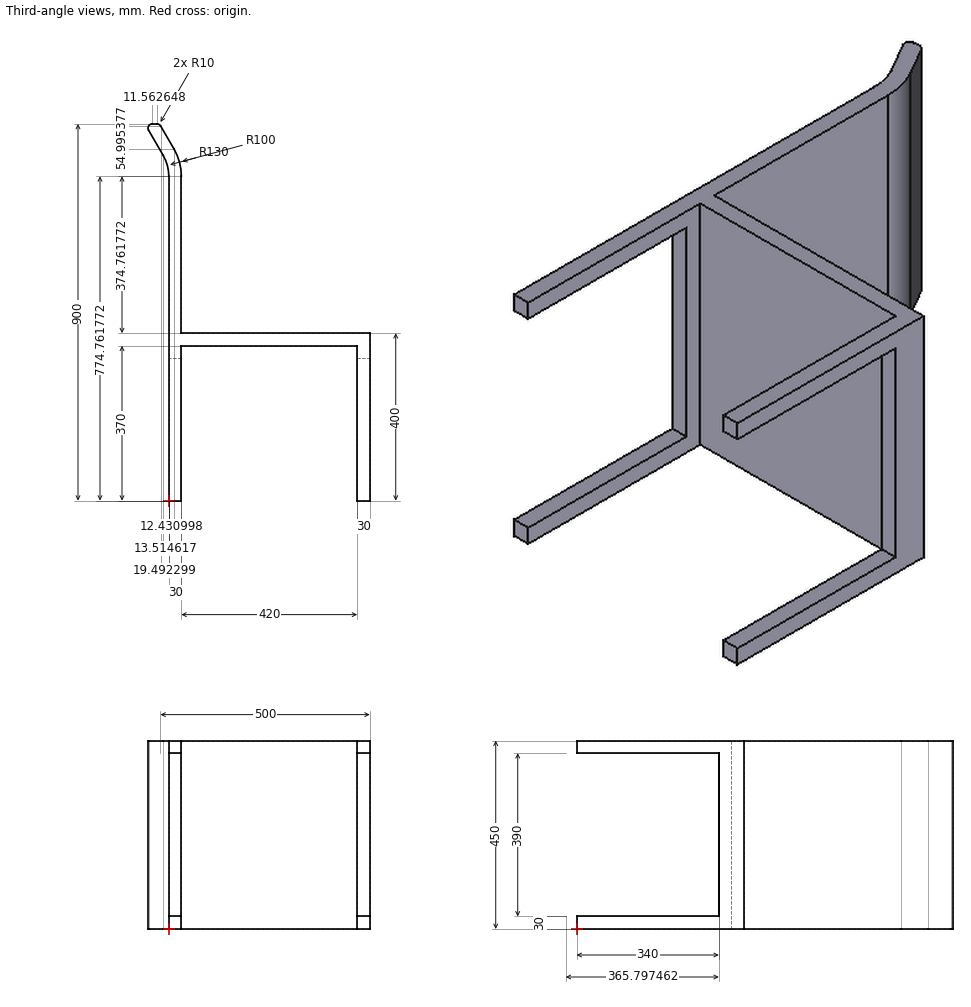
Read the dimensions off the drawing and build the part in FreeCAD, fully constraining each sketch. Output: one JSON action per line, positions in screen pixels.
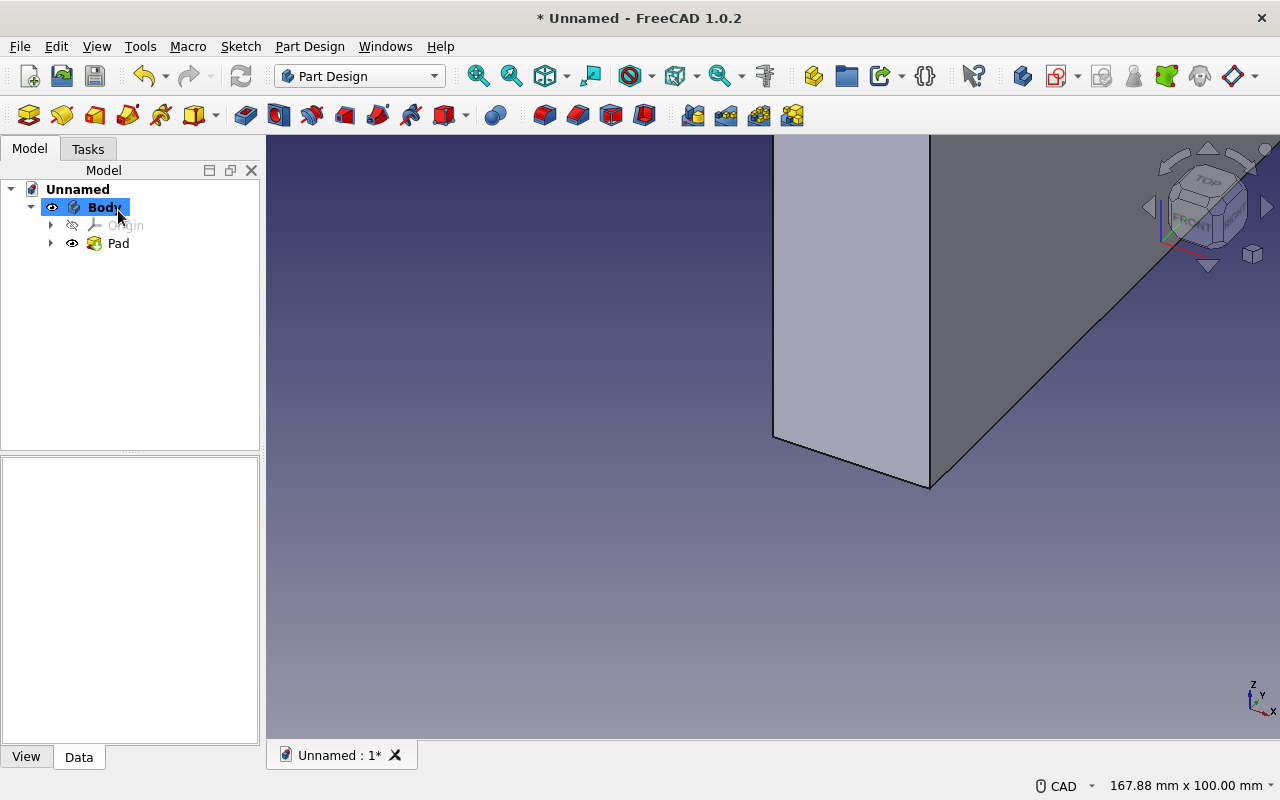
{"action": "key", "text": "v f"}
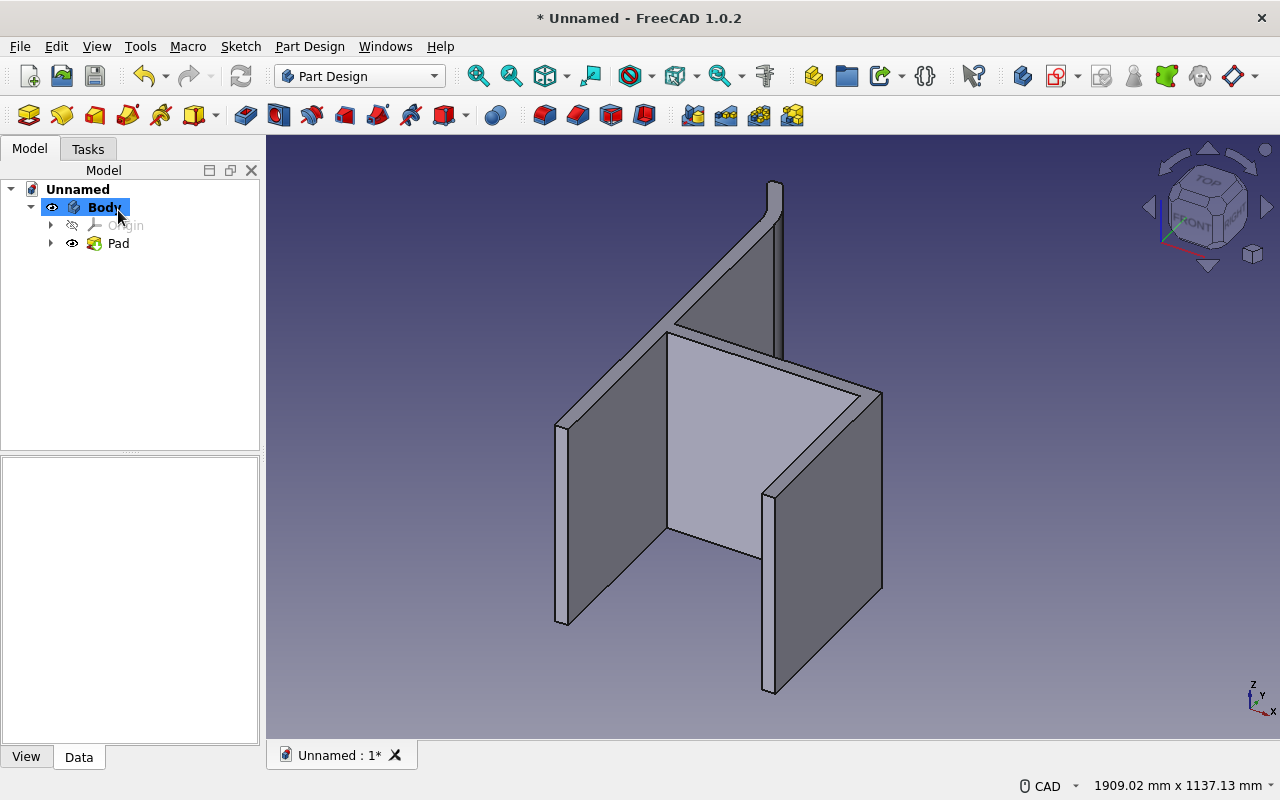
{"action": "left_click", "coordinate": [828, 542]}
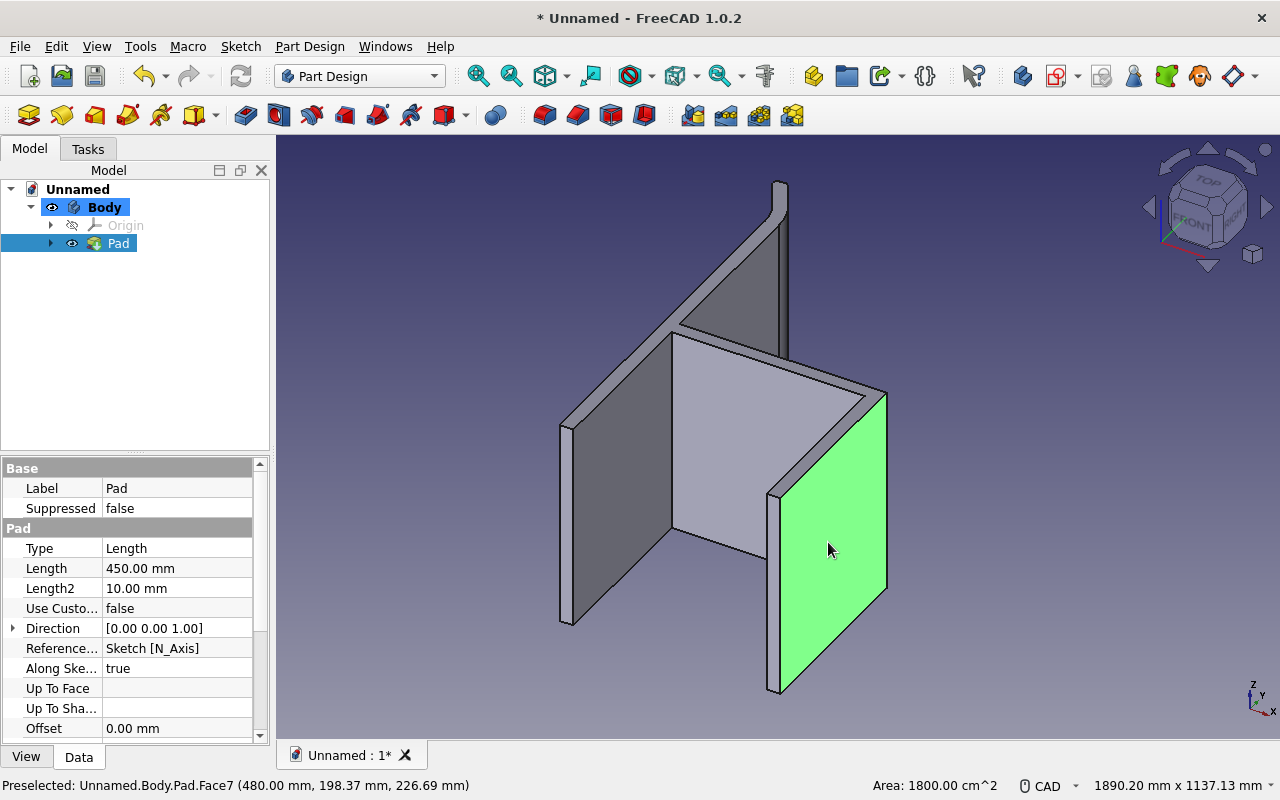
{"action": "left_click", "coordinate": [1056, 76]}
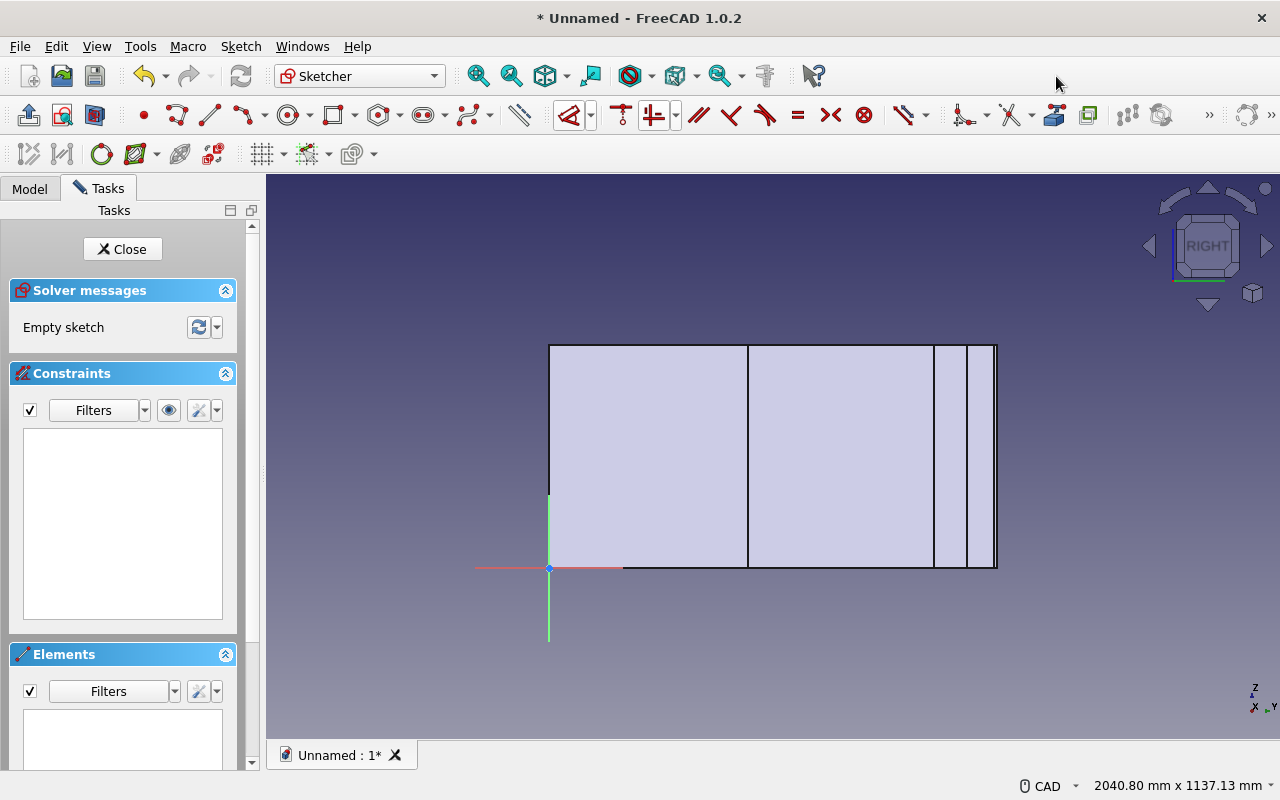
{"action": "scroll", "coordinate": [534, 473], "scroll_direction": "up", "scroll_amount": 3}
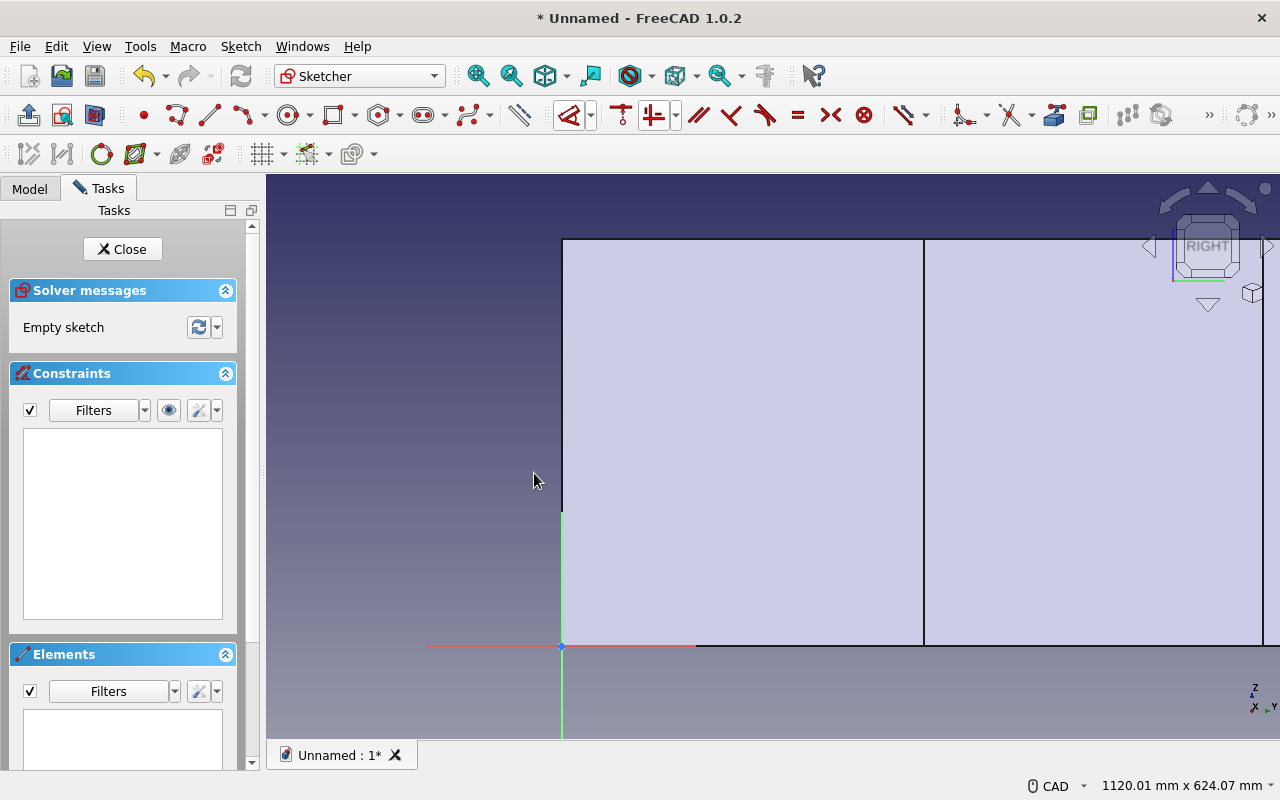
{"action": "left_click", "coordinate": [332, 116]}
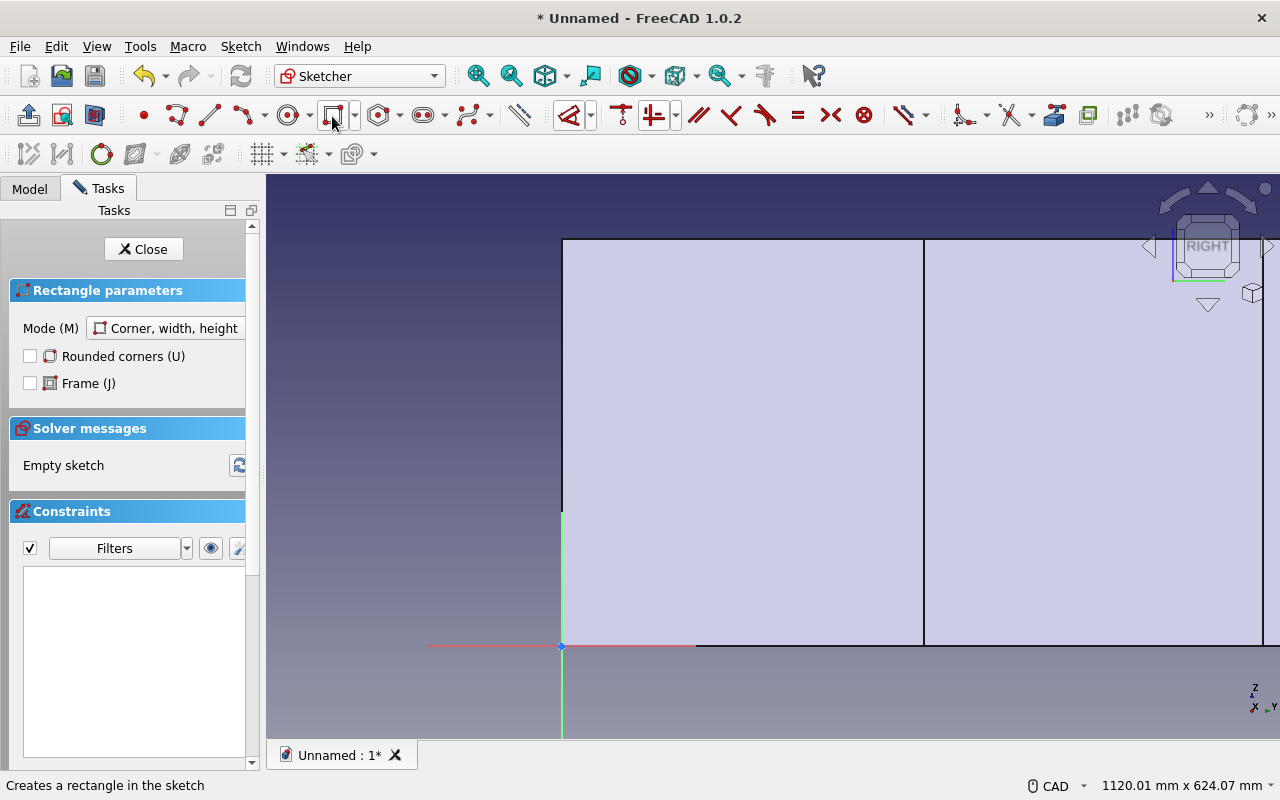
{"action": "left_click", "coordinate": [539, 266]}
{"action": "left_click", "coordinate": [870, 619]}
{"action": "key", "text": "Escape"}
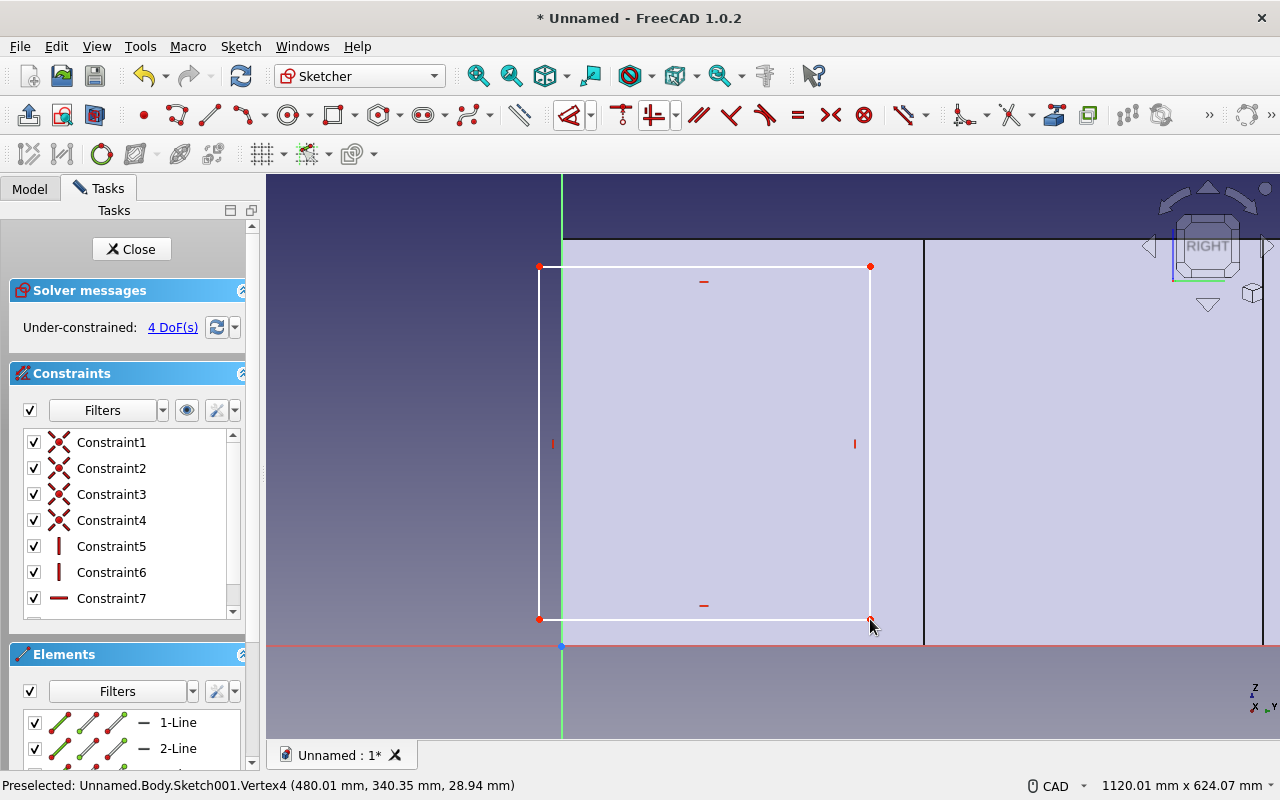
{"action": "left_click", "coordinate": [539, 373]}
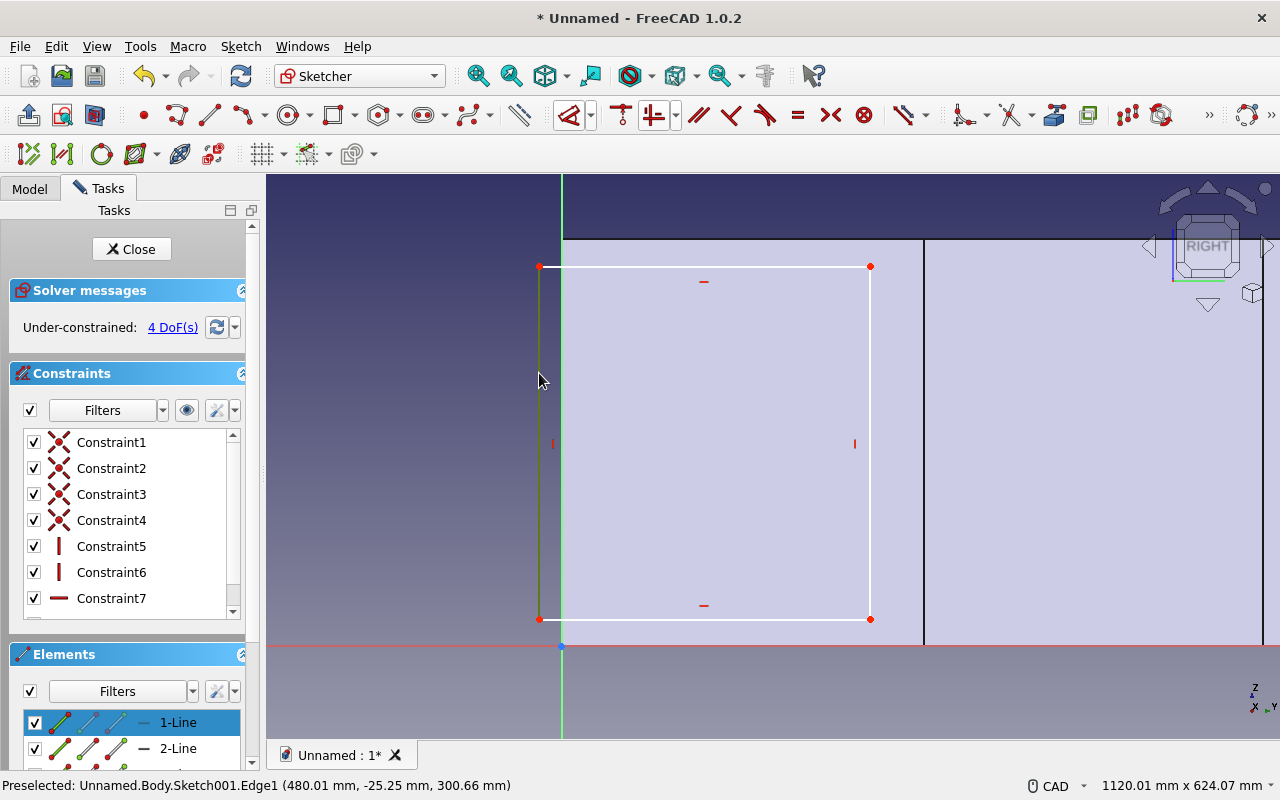
{"action": "key", "text": "i"}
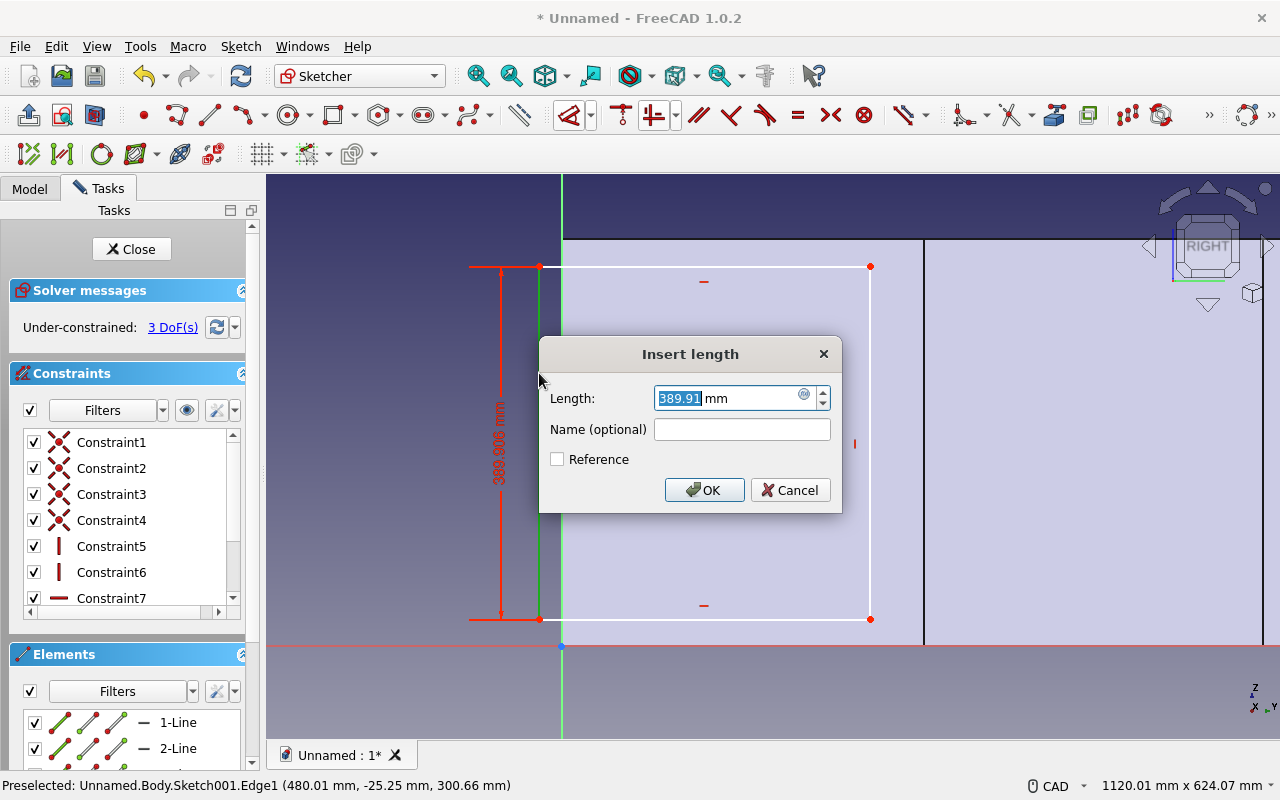
{"action": "type", "text": "390"}
{"action": "key", "text": "Return"}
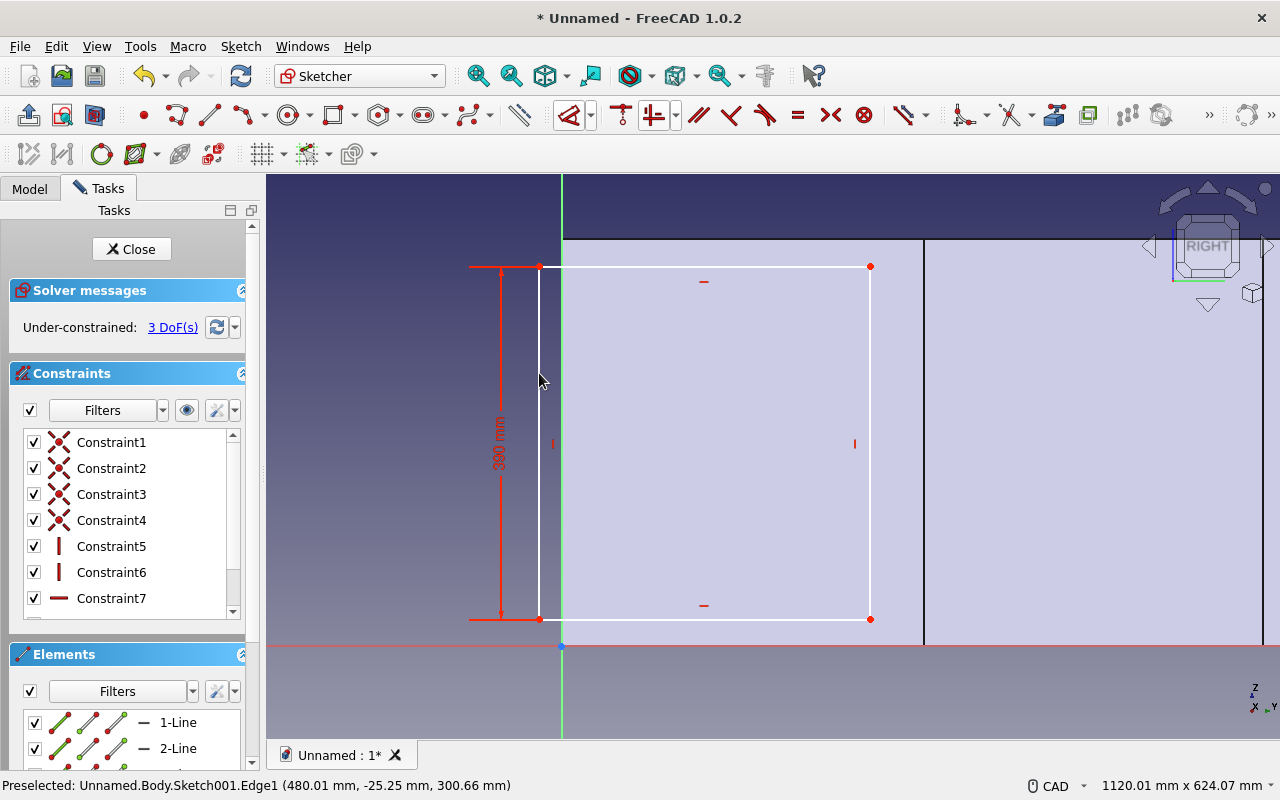
{"action": "scroll", "coordinate": [539, 620], "scroll_direction": "up", "scroll_amount": 2}